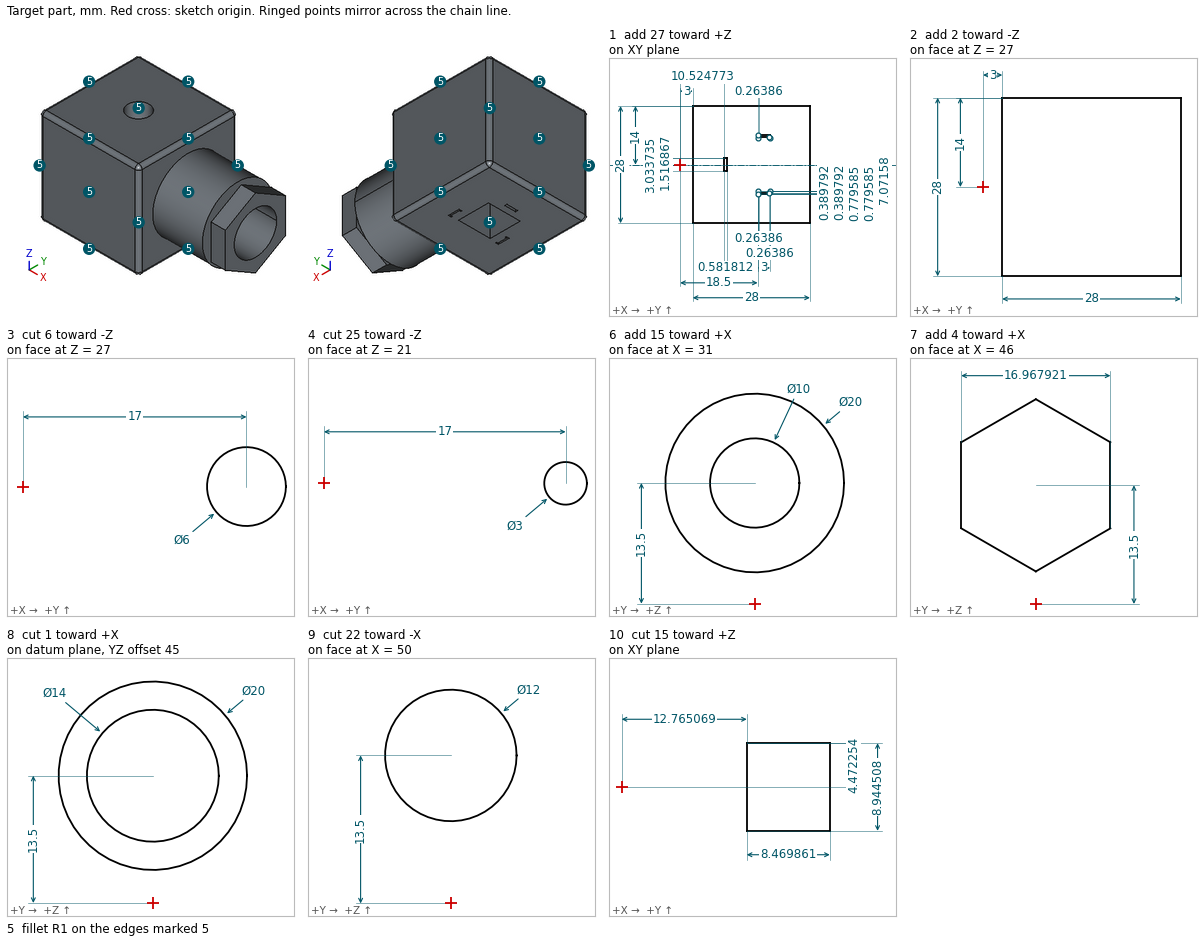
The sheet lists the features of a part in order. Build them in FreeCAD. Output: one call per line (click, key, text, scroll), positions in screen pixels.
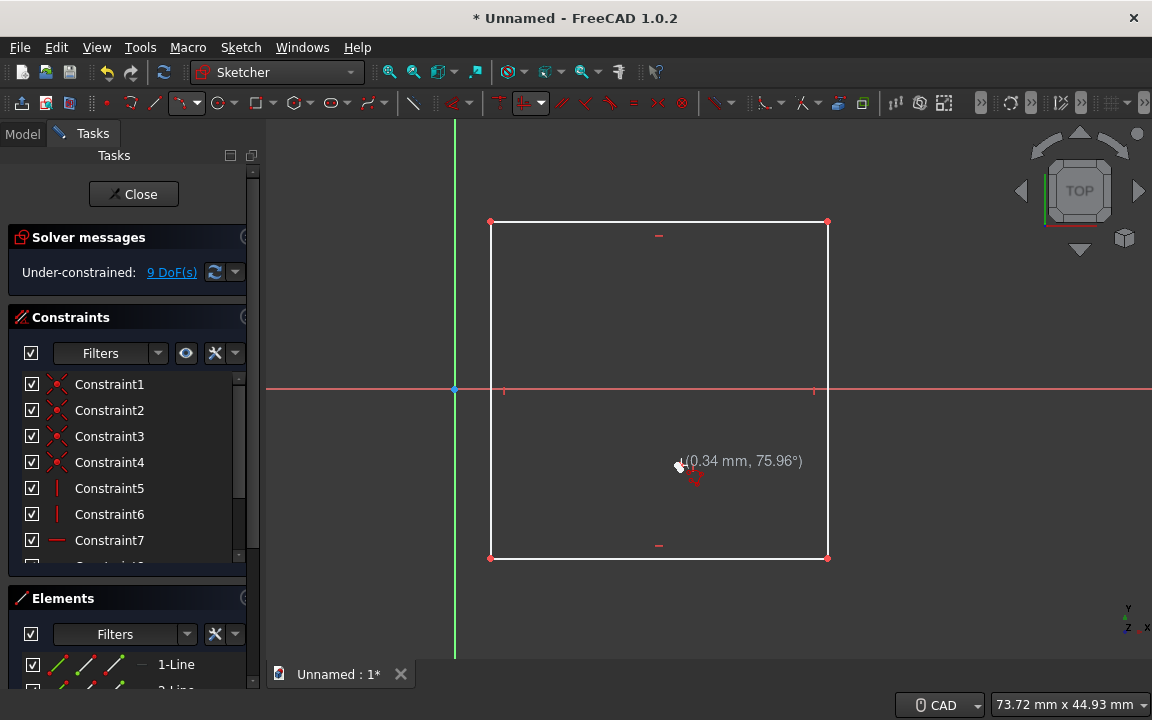
click(710, 470)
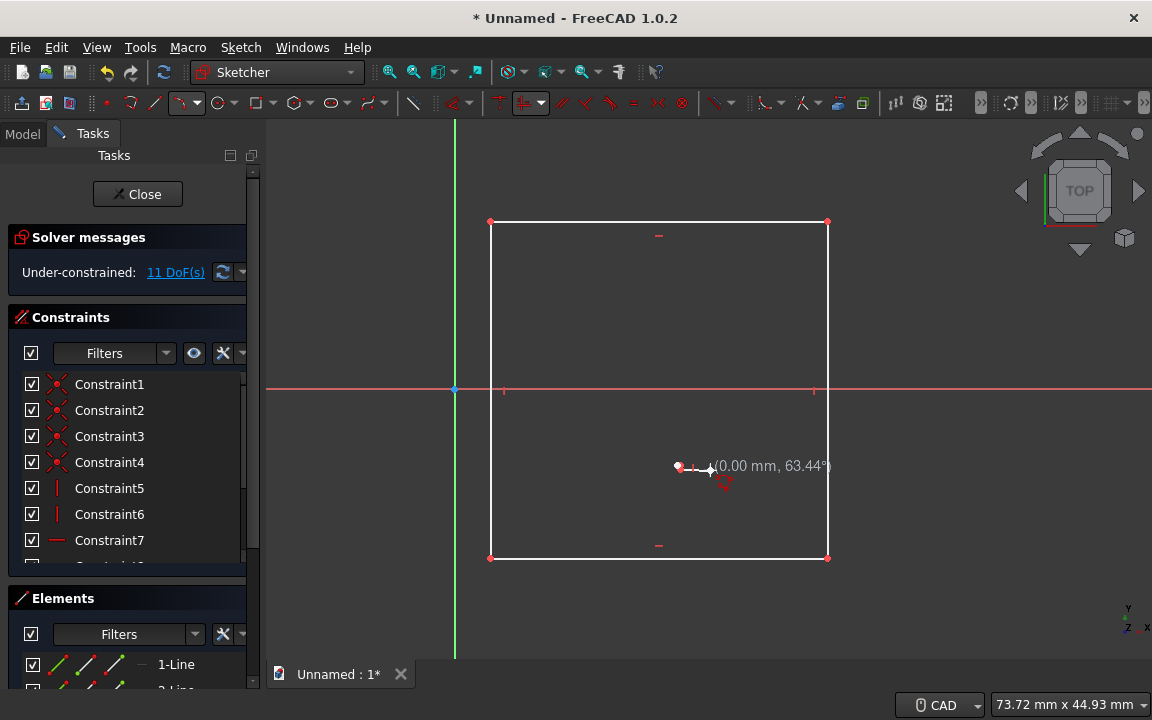
scroll(710, 465, up, 7)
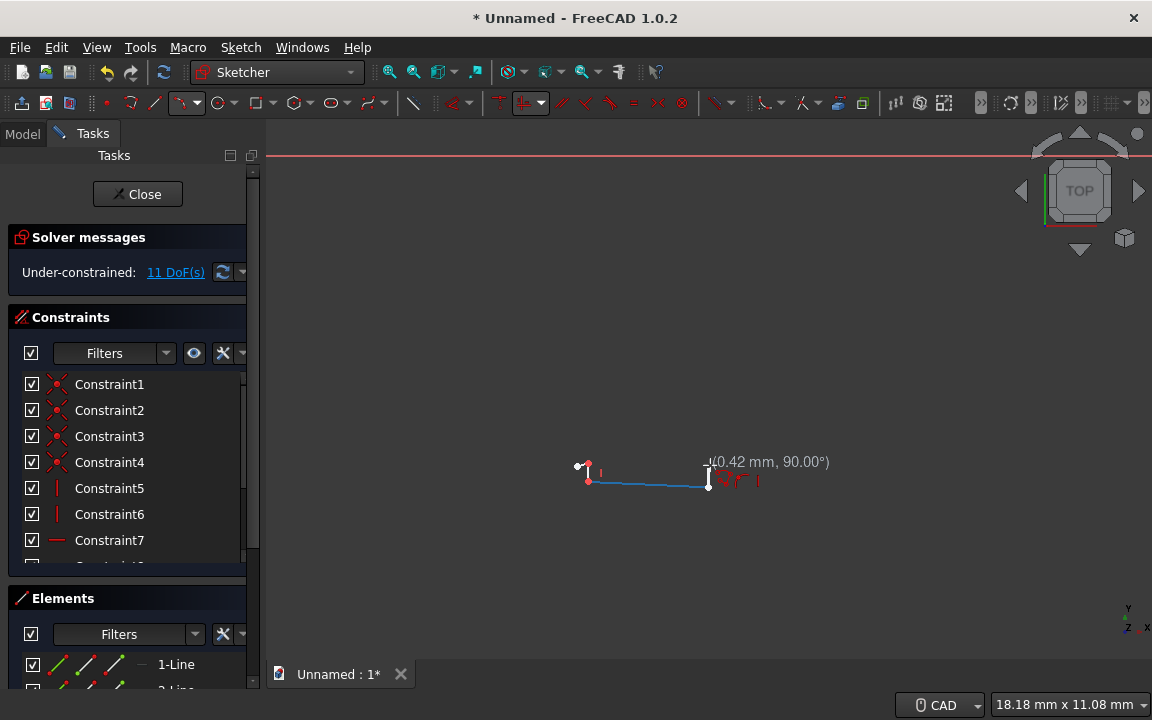
click(708, 462)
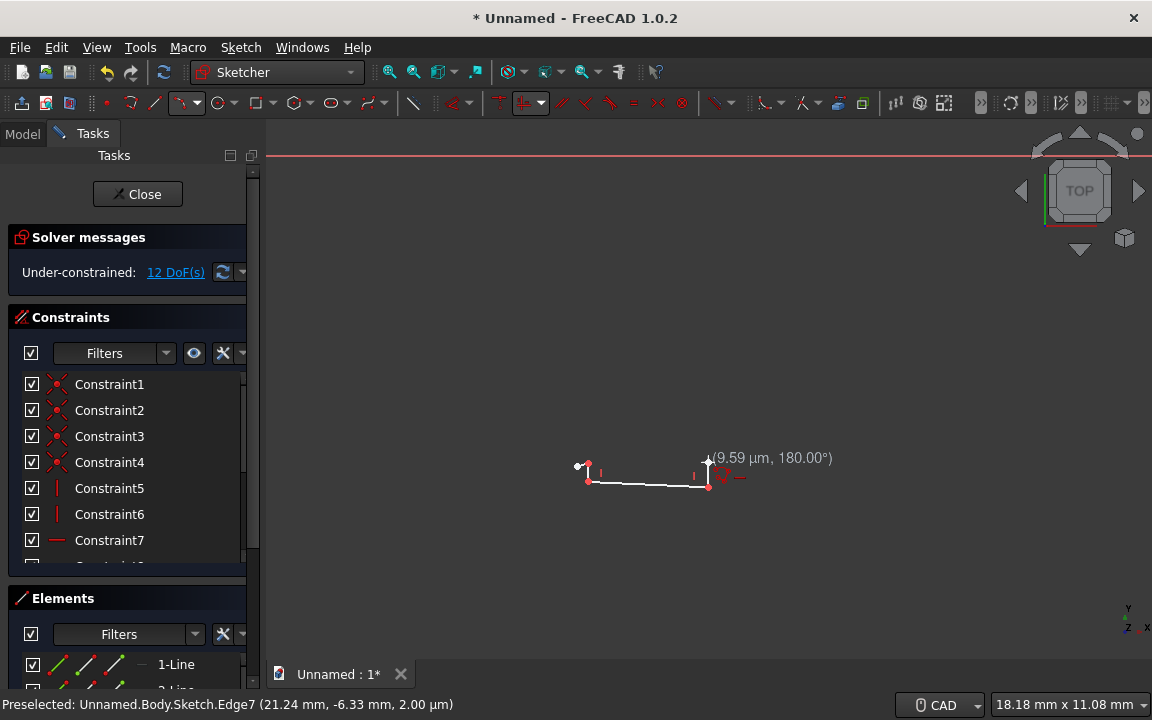
scroll(722, 462, up, 2)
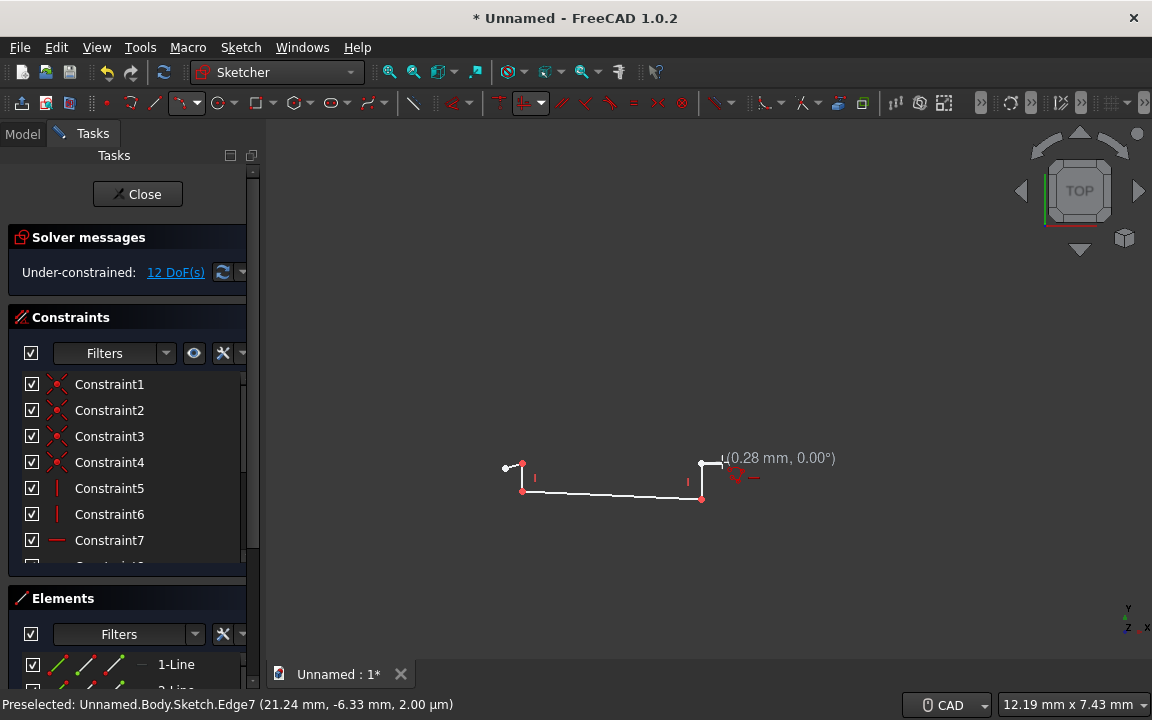
click(721, 462)
click(721, 519)
click(503, 519)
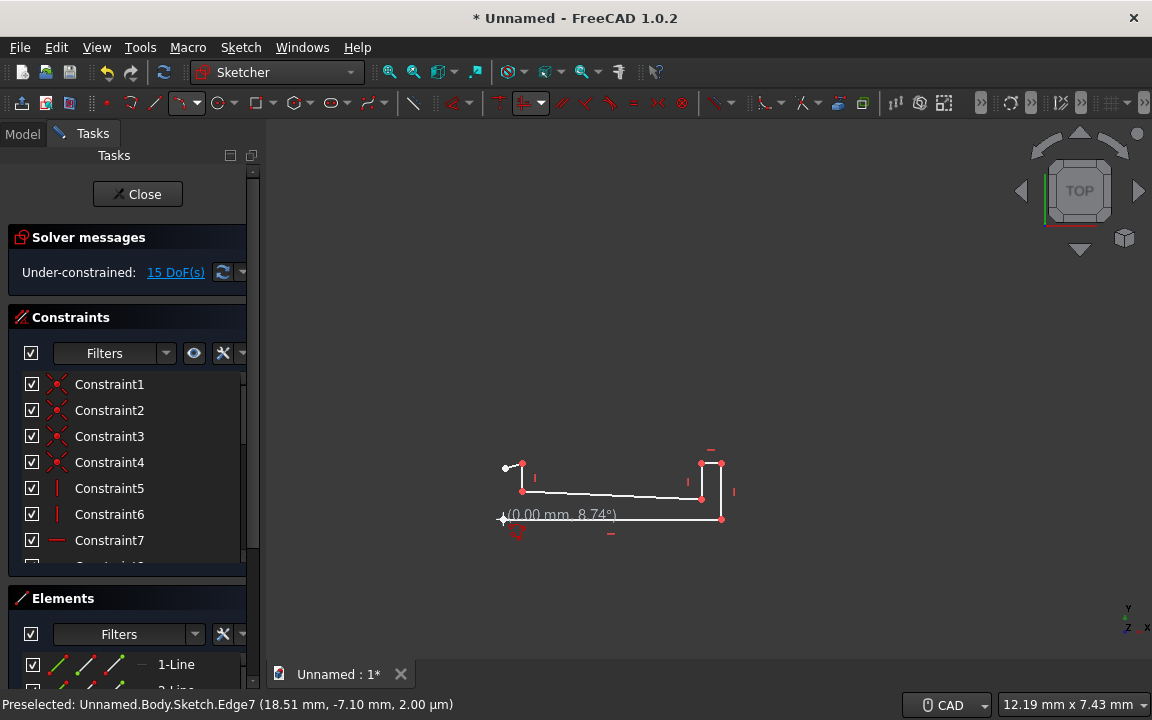
scroll(503, 462, up, 3)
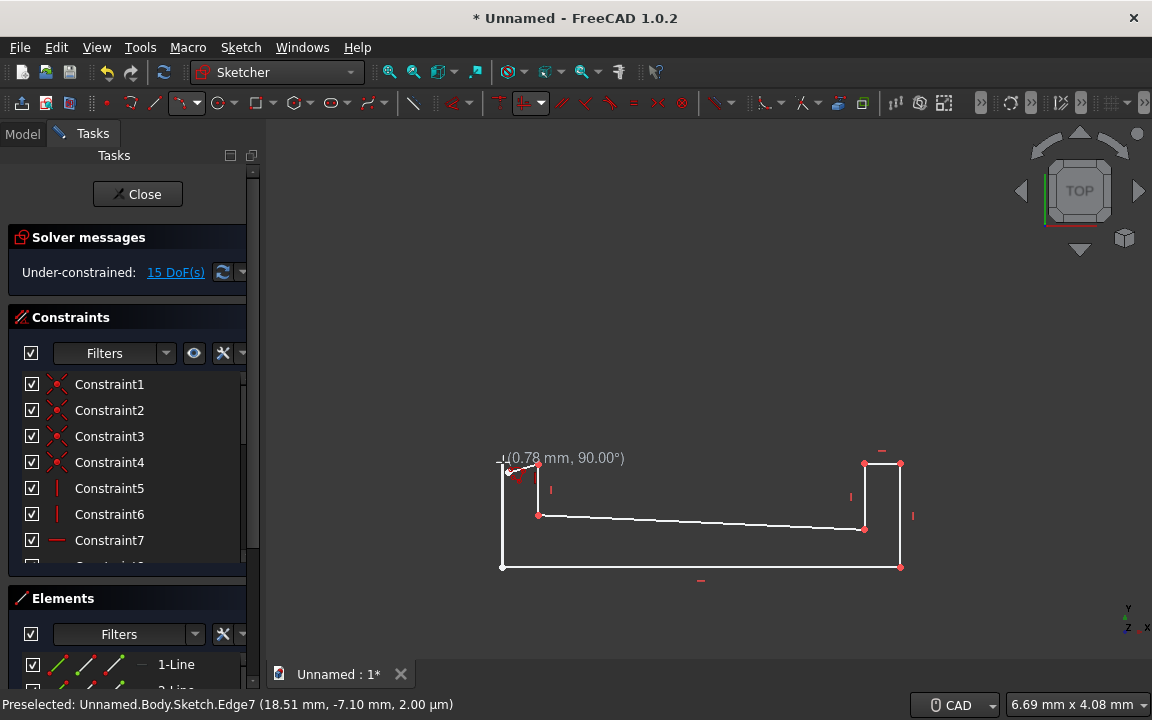
click(508, 462)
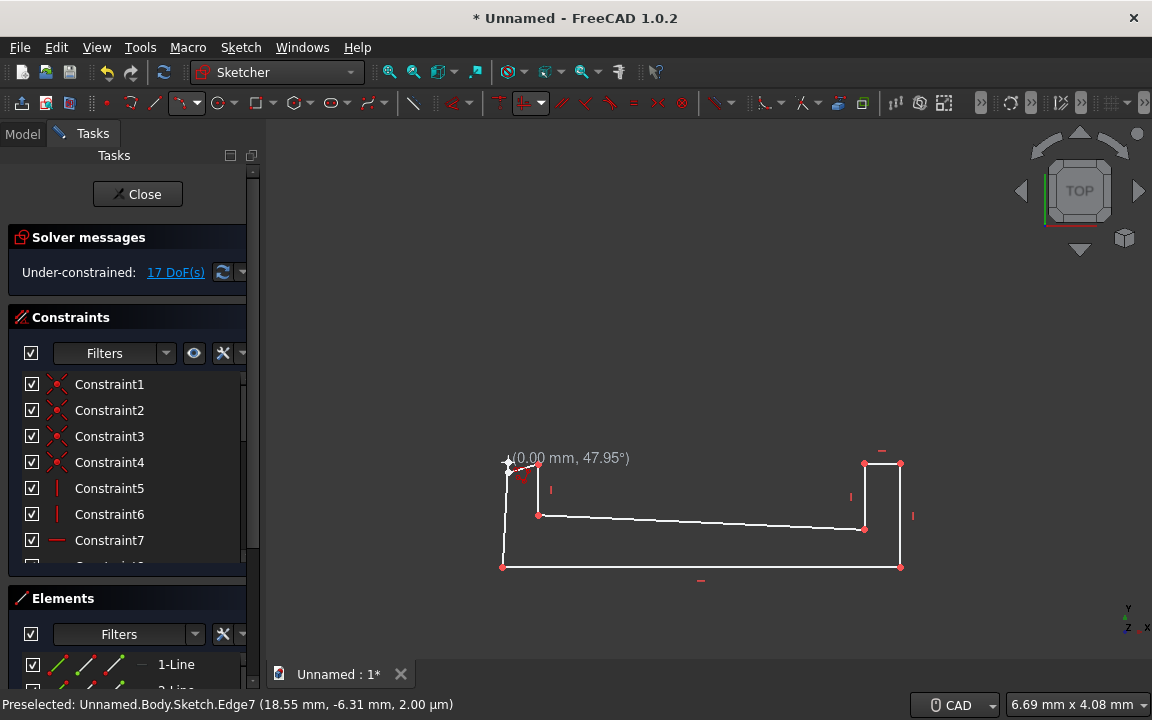
click(256, 104)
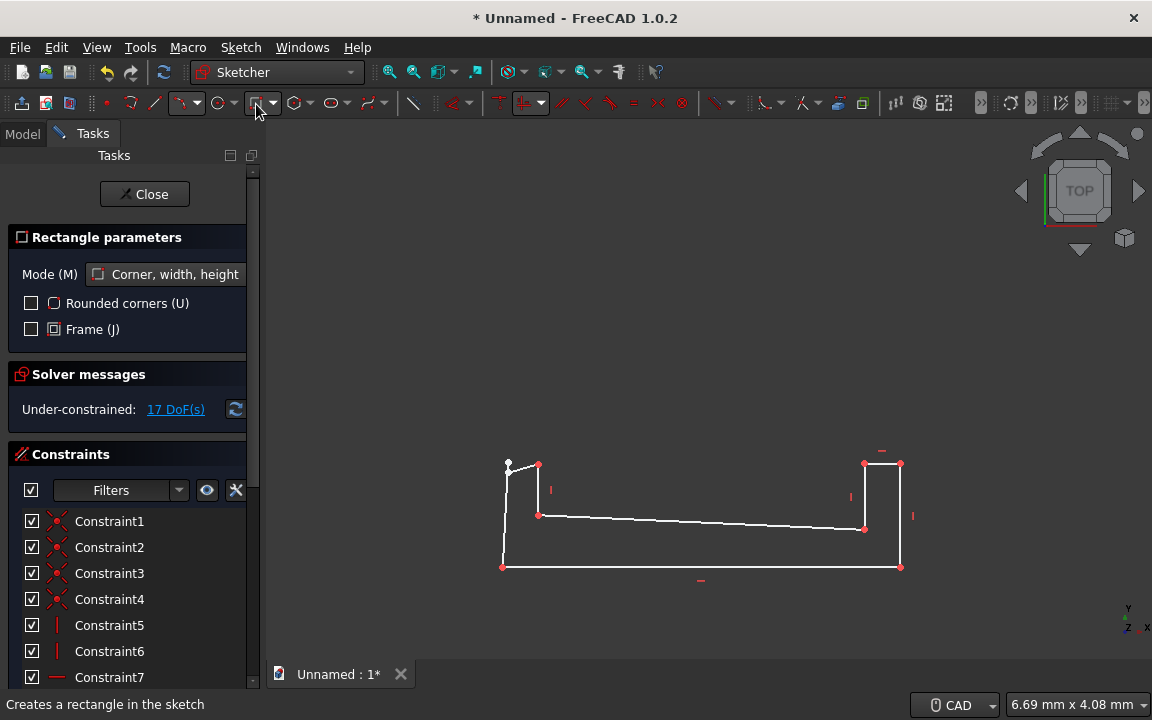
scroll(694, 465, down, 12)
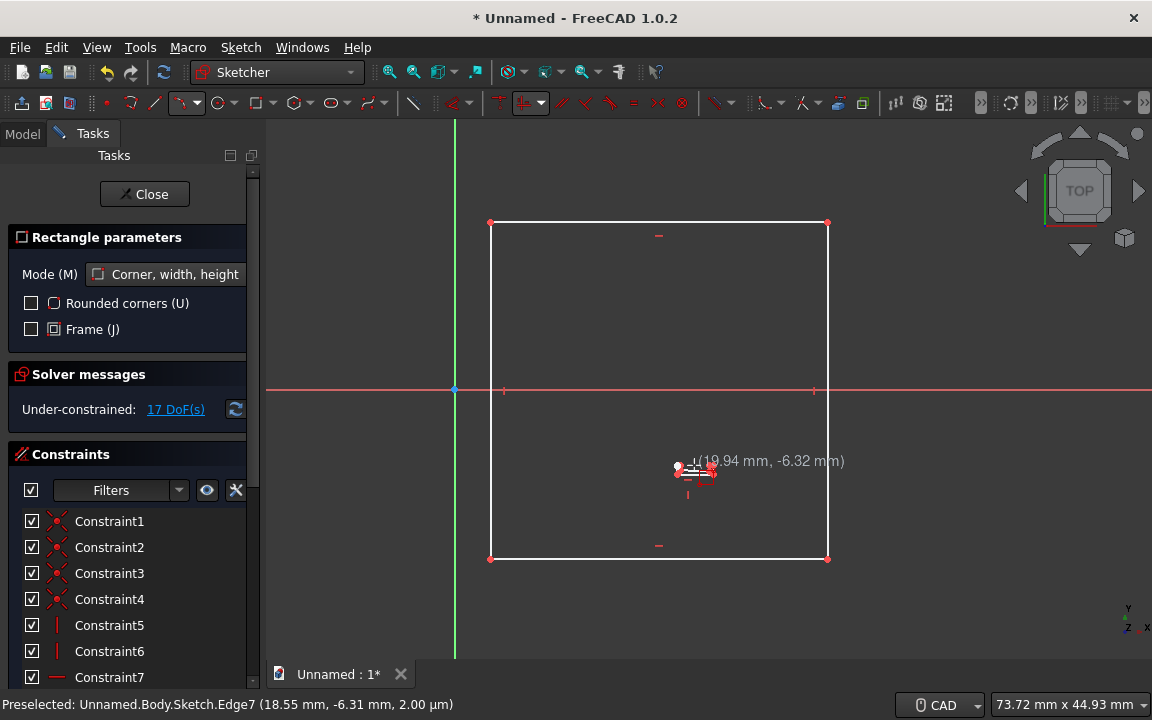
scroll(581, 371, up, 5)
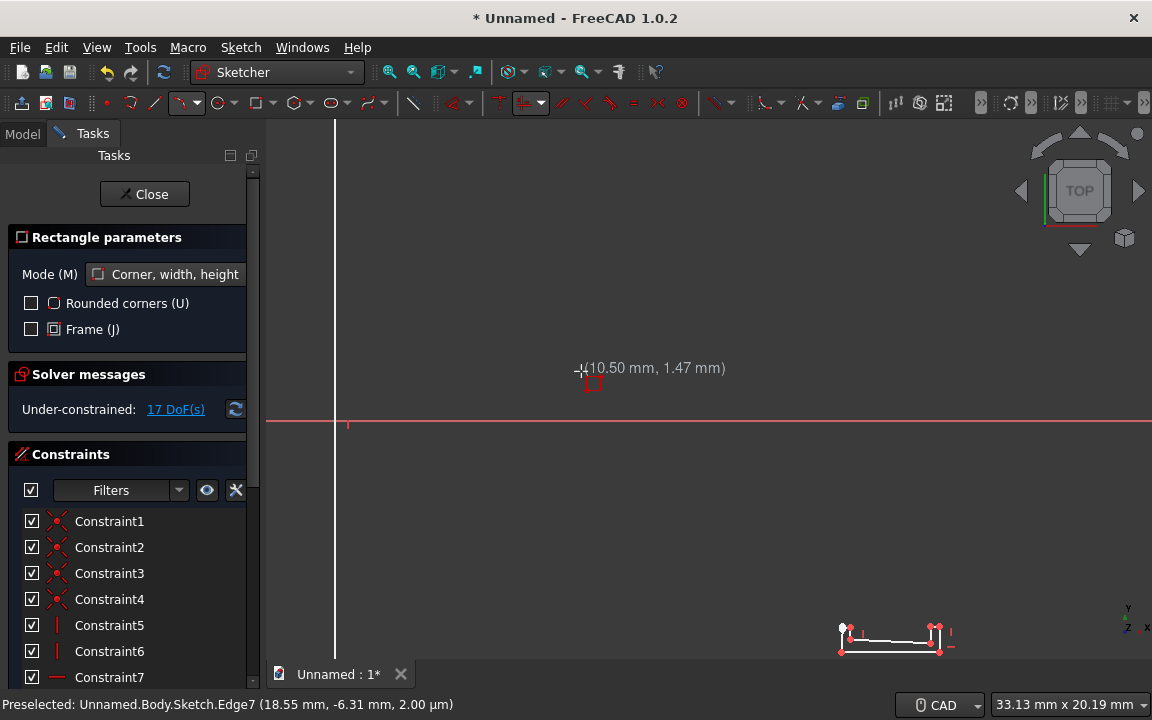
click(581, 371)
click(600, 471)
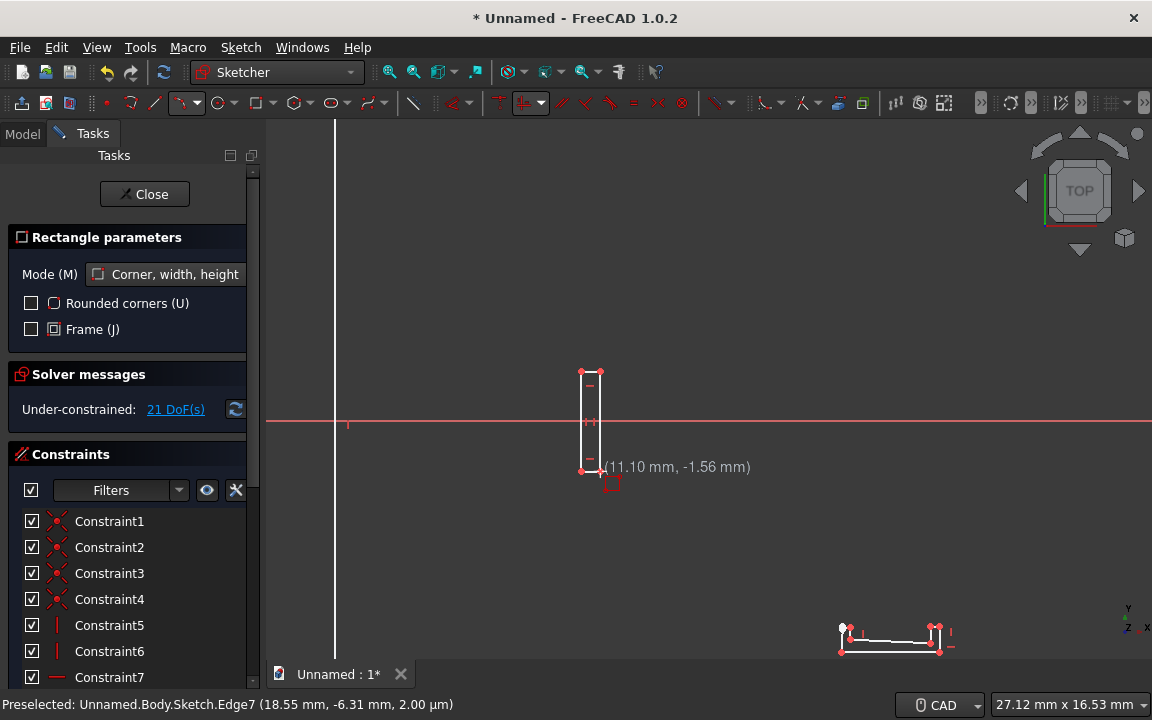
click(132, 104)